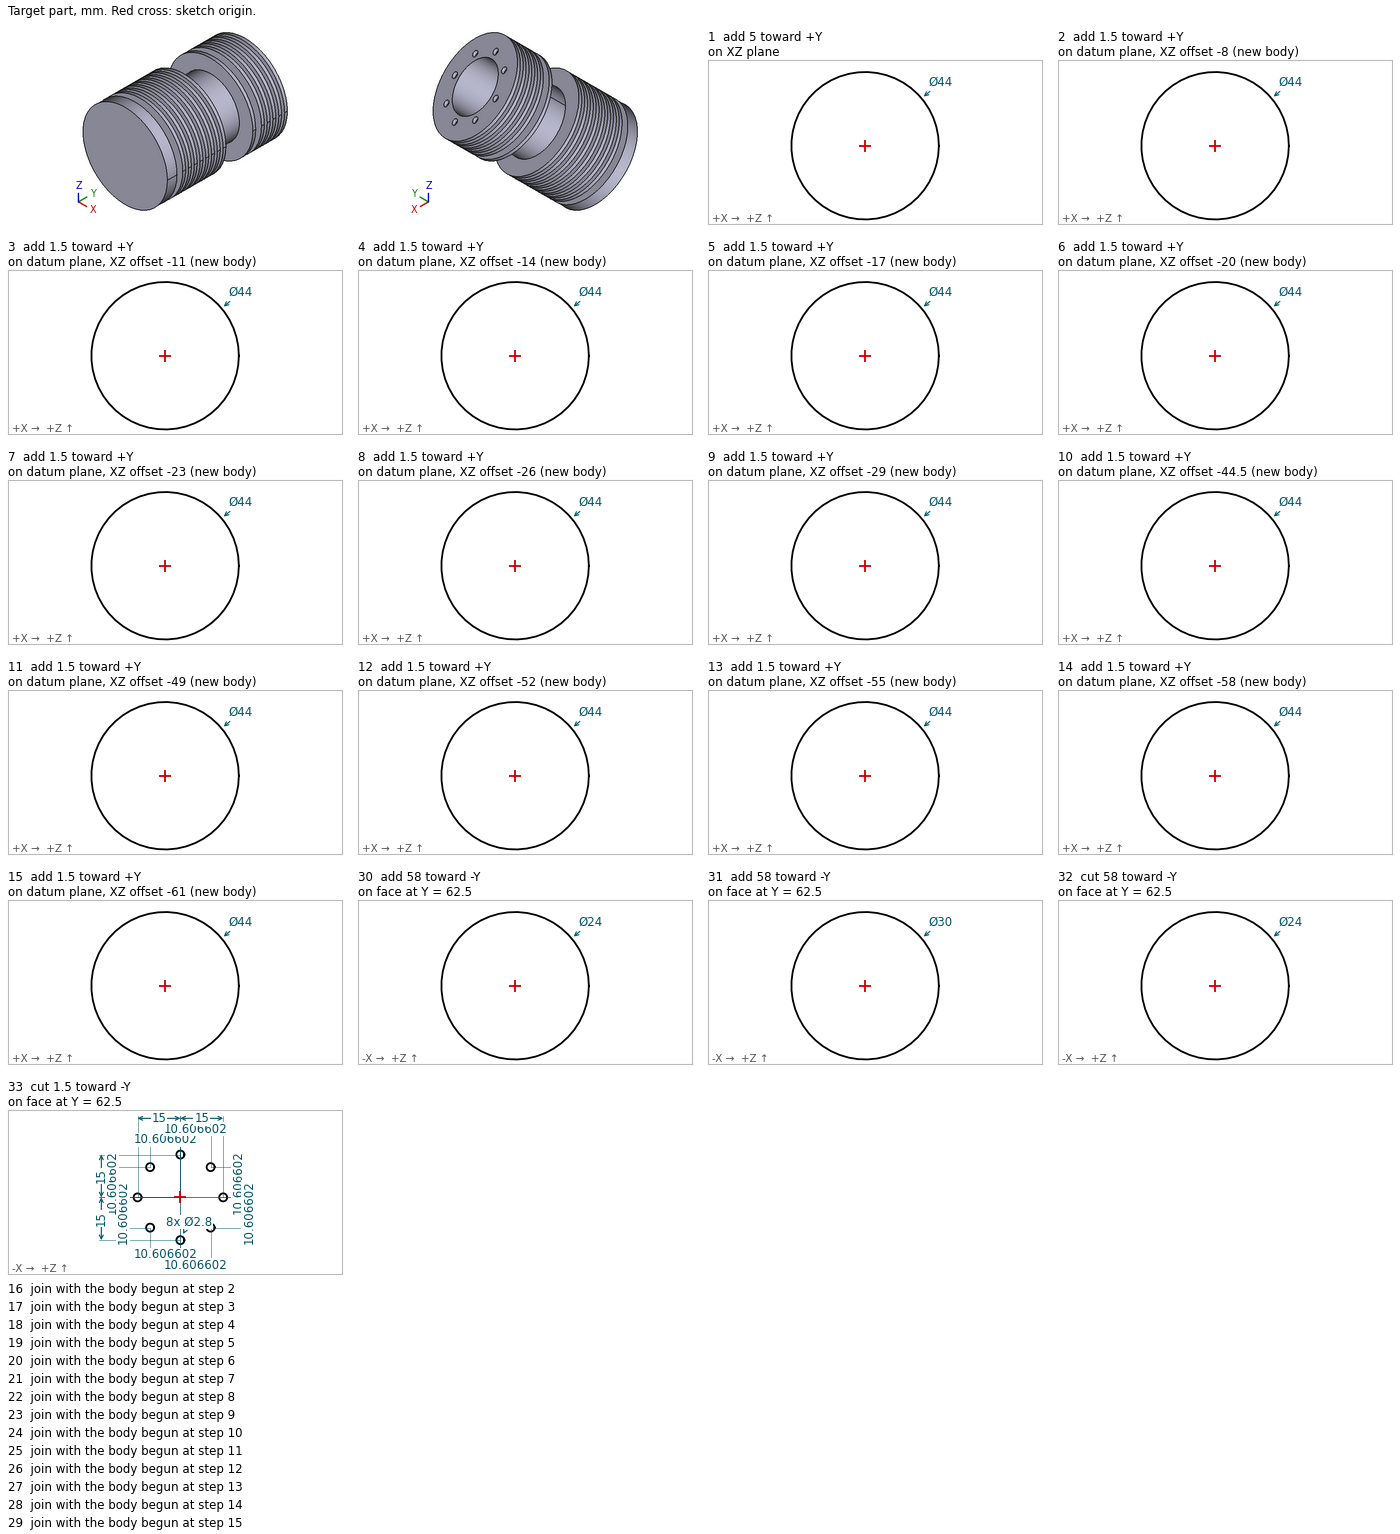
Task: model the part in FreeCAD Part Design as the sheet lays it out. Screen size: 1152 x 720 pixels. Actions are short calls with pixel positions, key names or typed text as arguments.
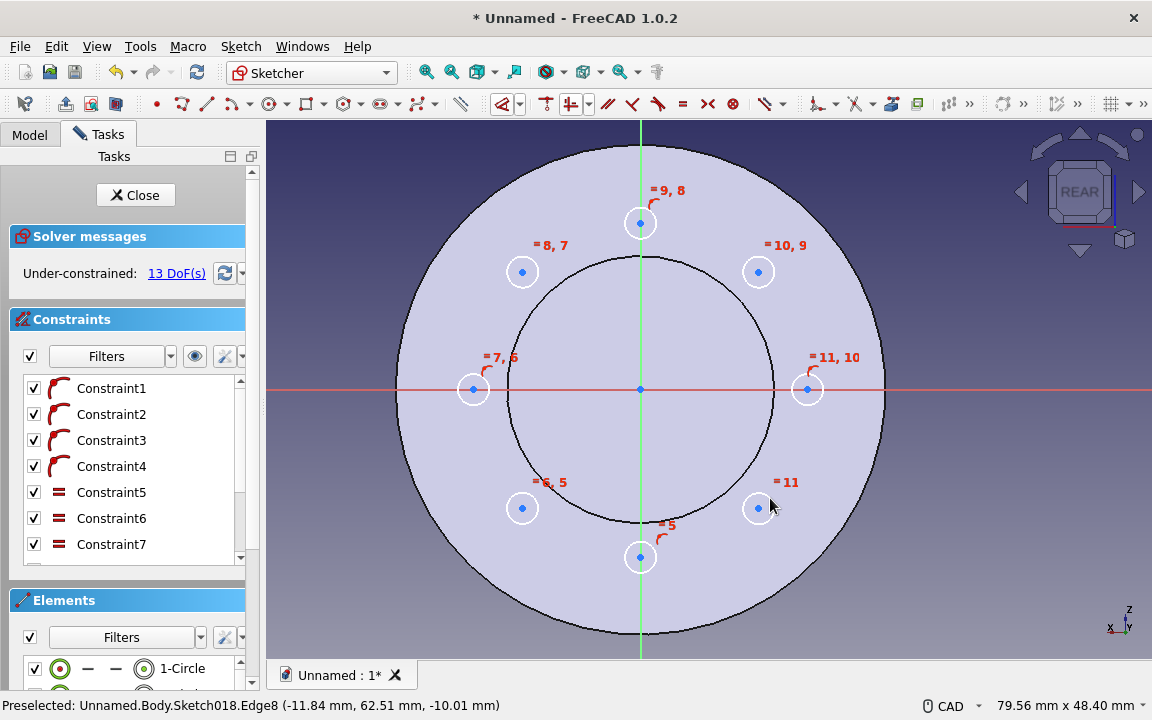
scroll(652, 546, up, 2)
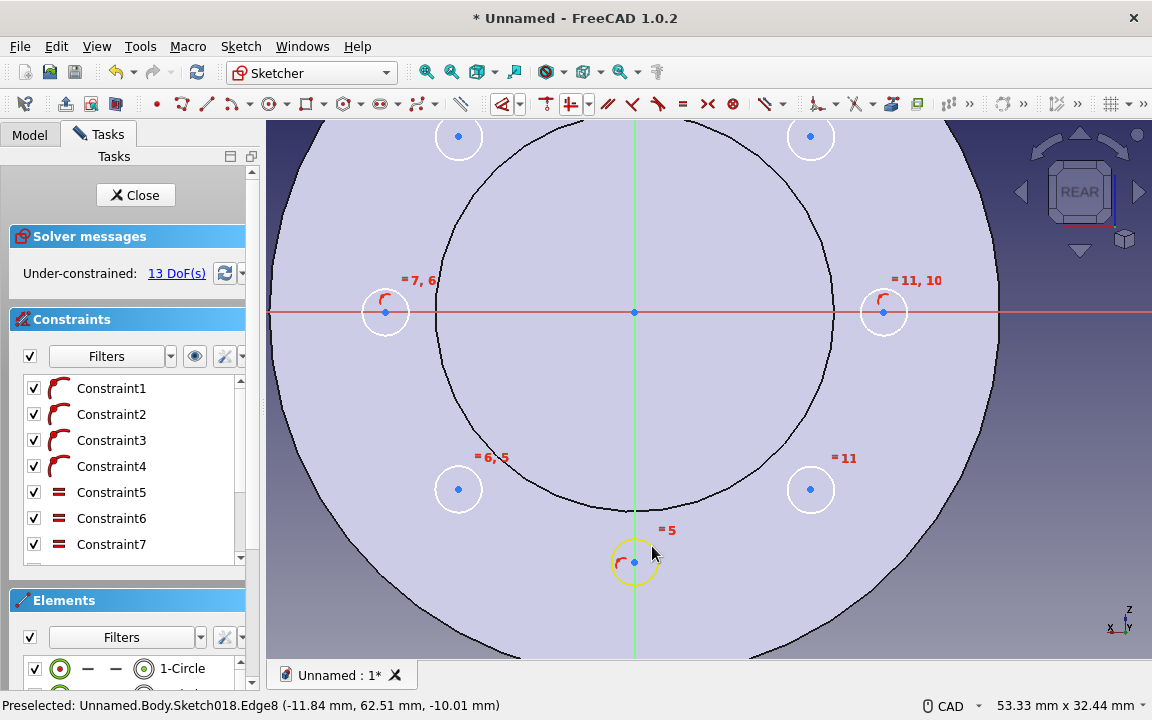
click(651, 546)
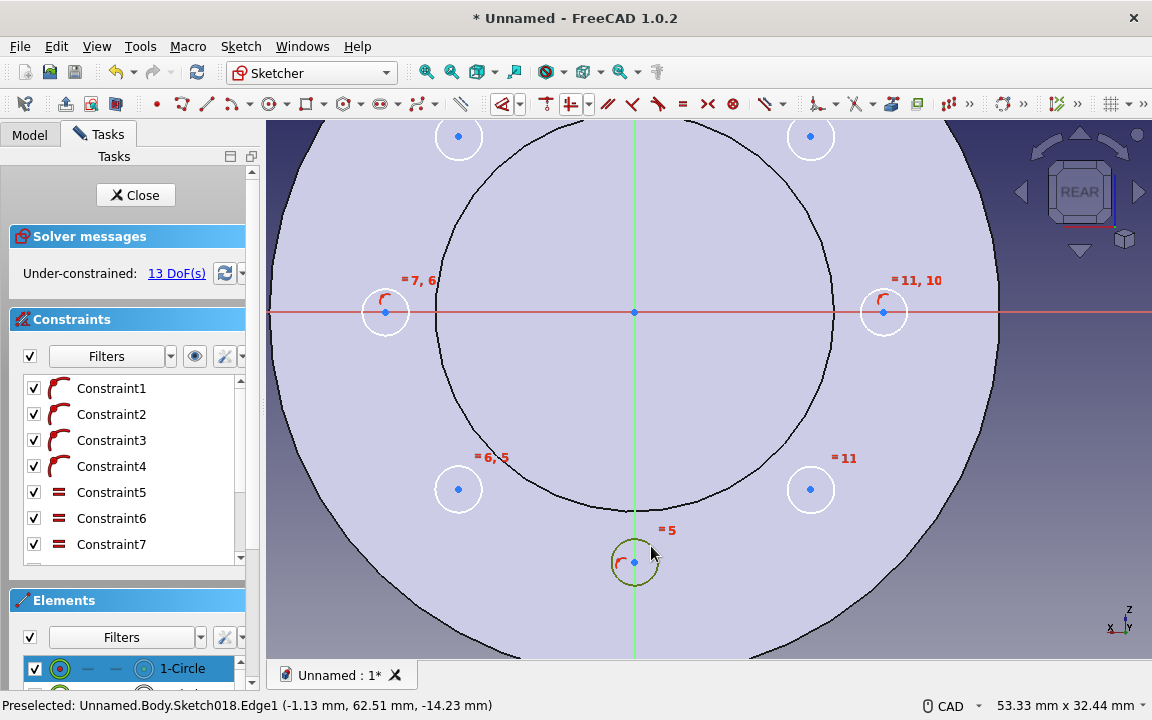
click(520, 104)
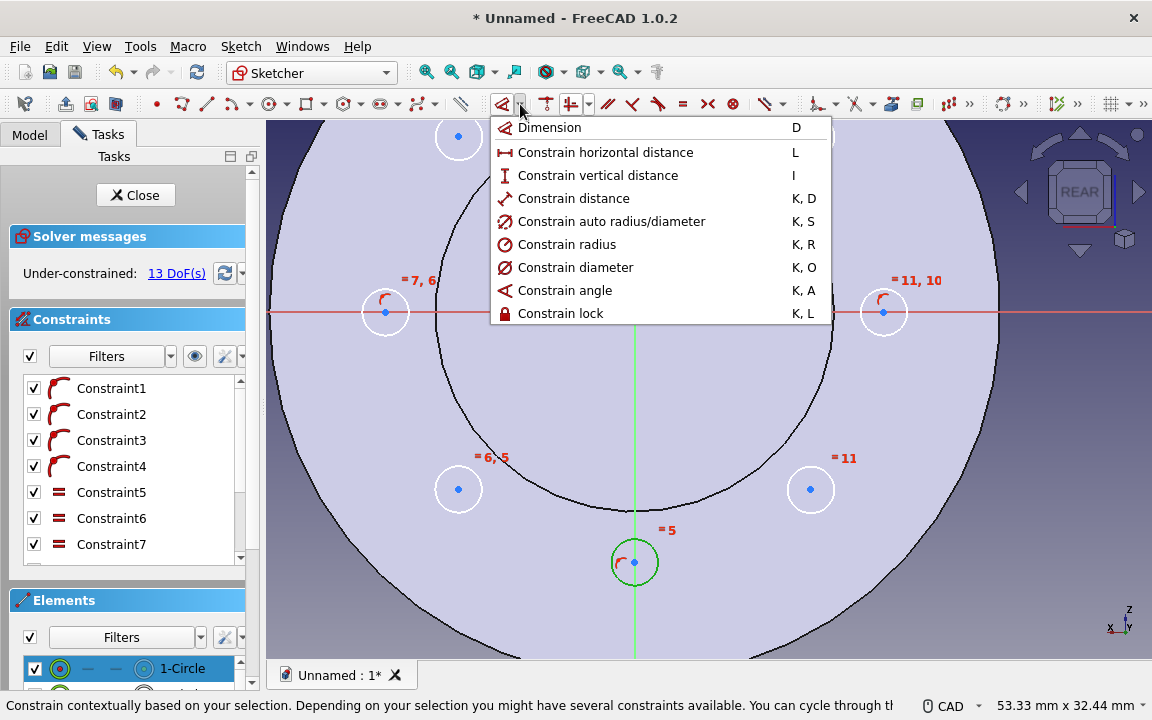
click(661, 268)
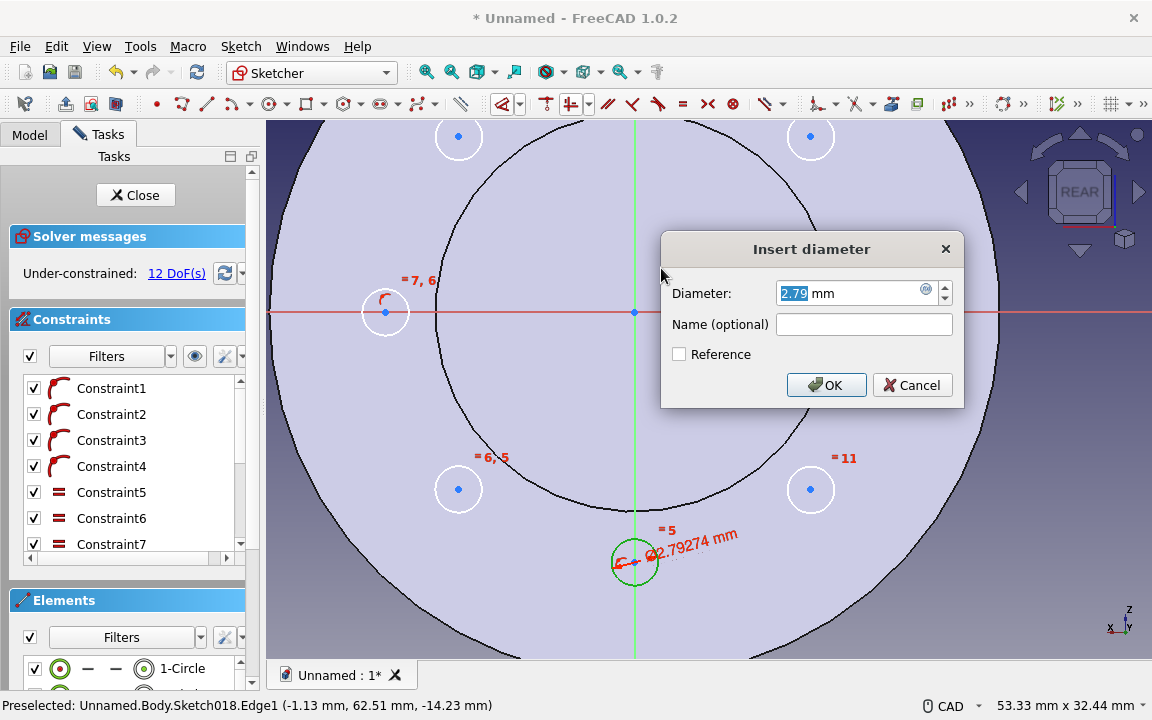
text(2.8)
key(Return)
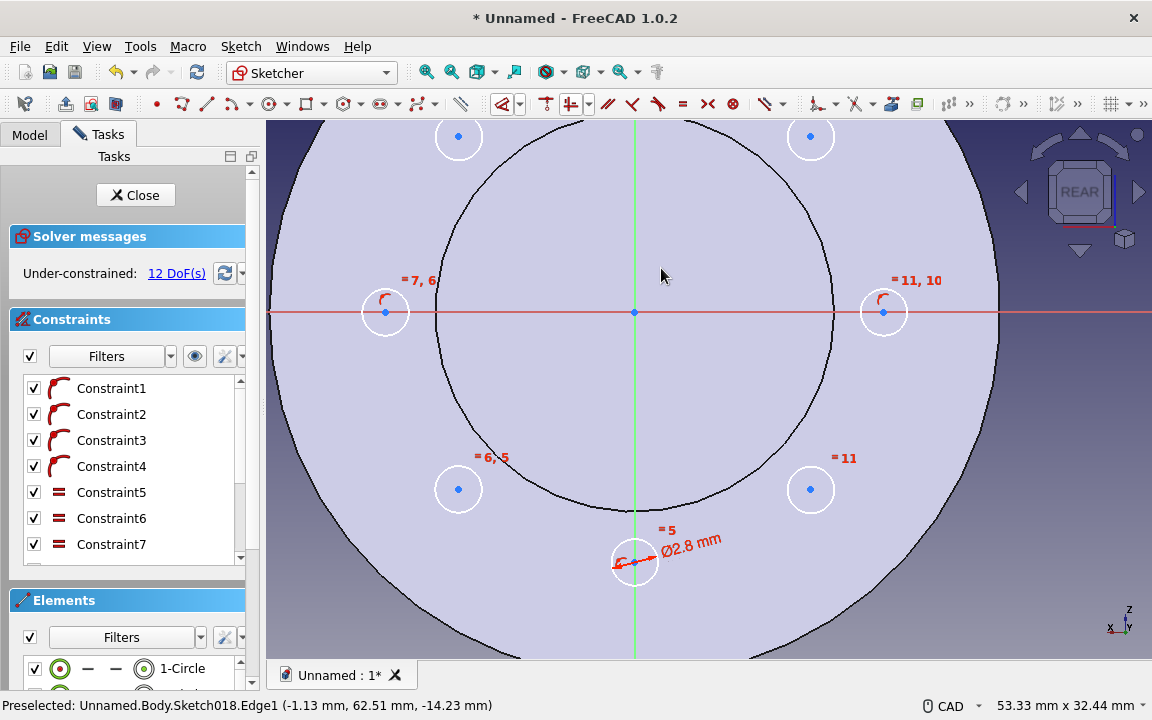
click(635, 562)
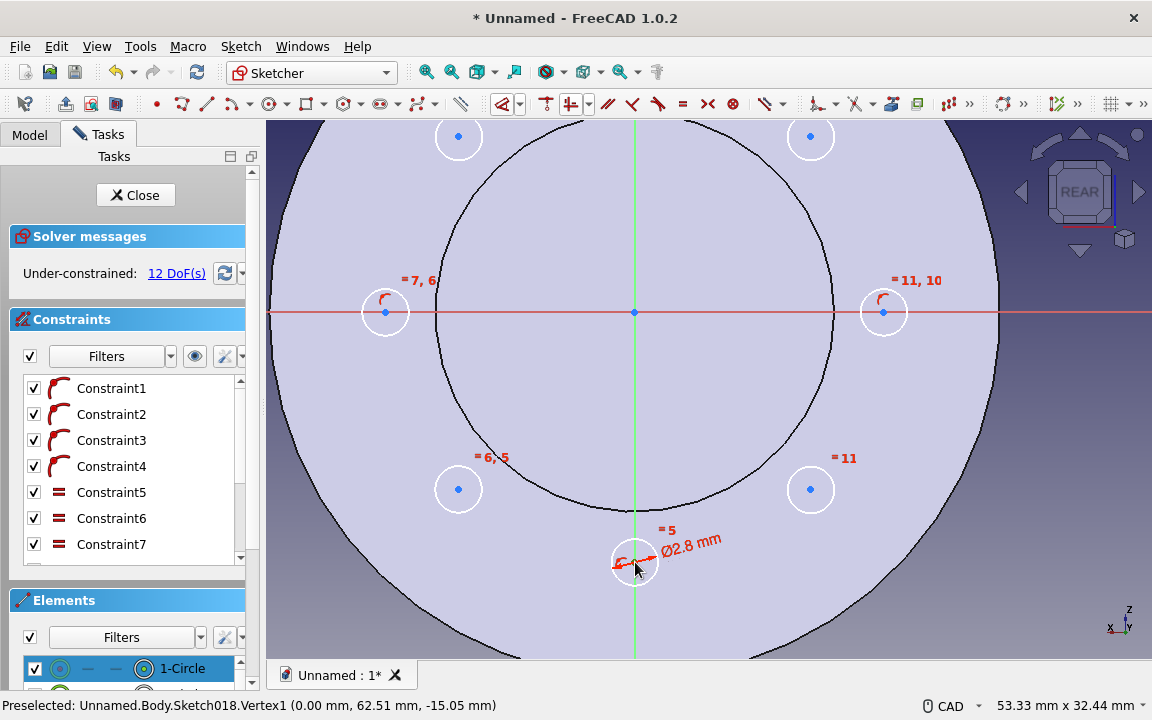
key(i)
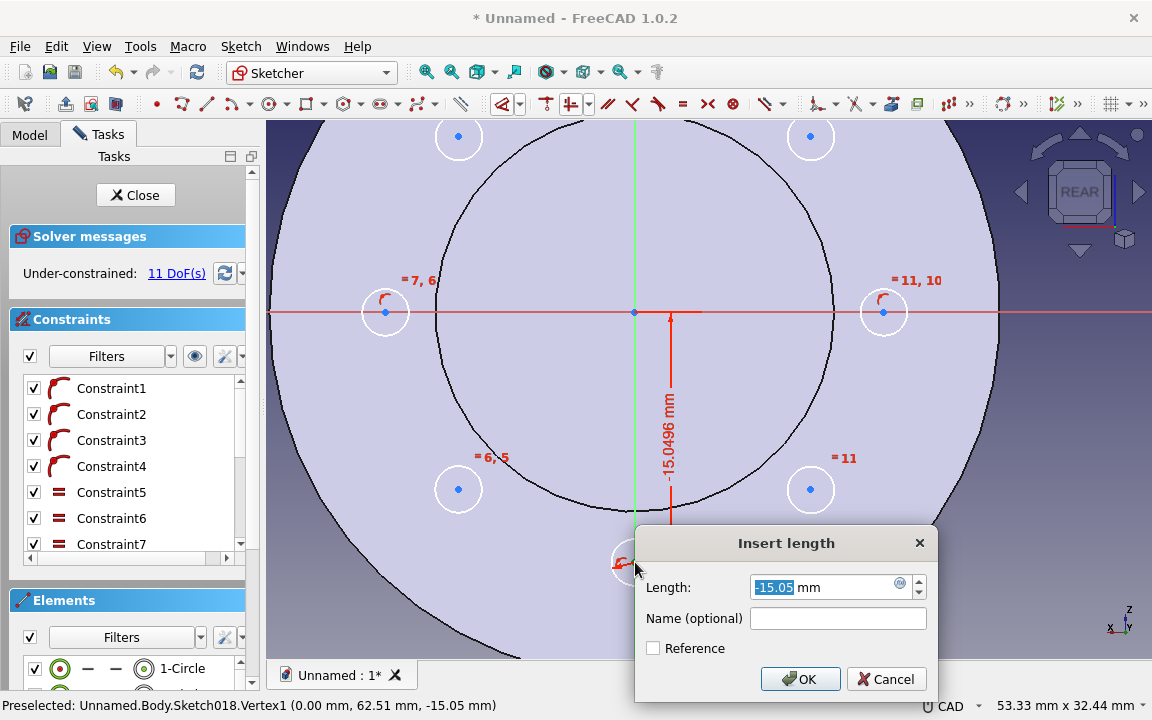
text(-15)
key(Return)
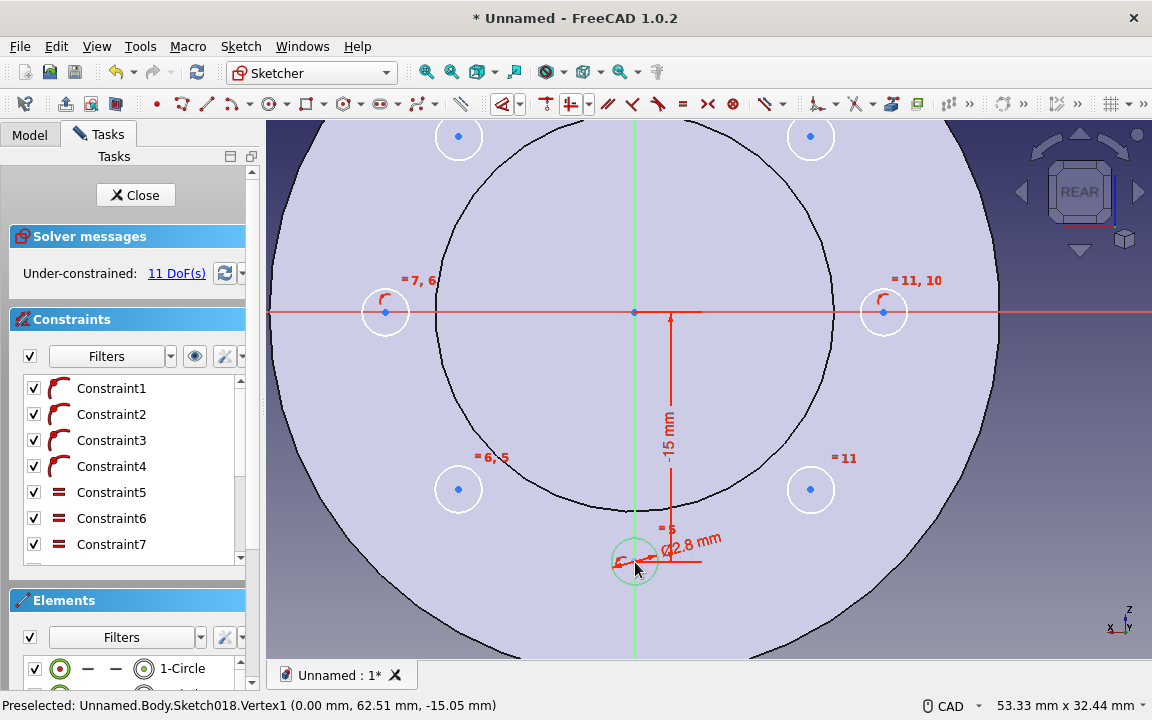
click(386, 312)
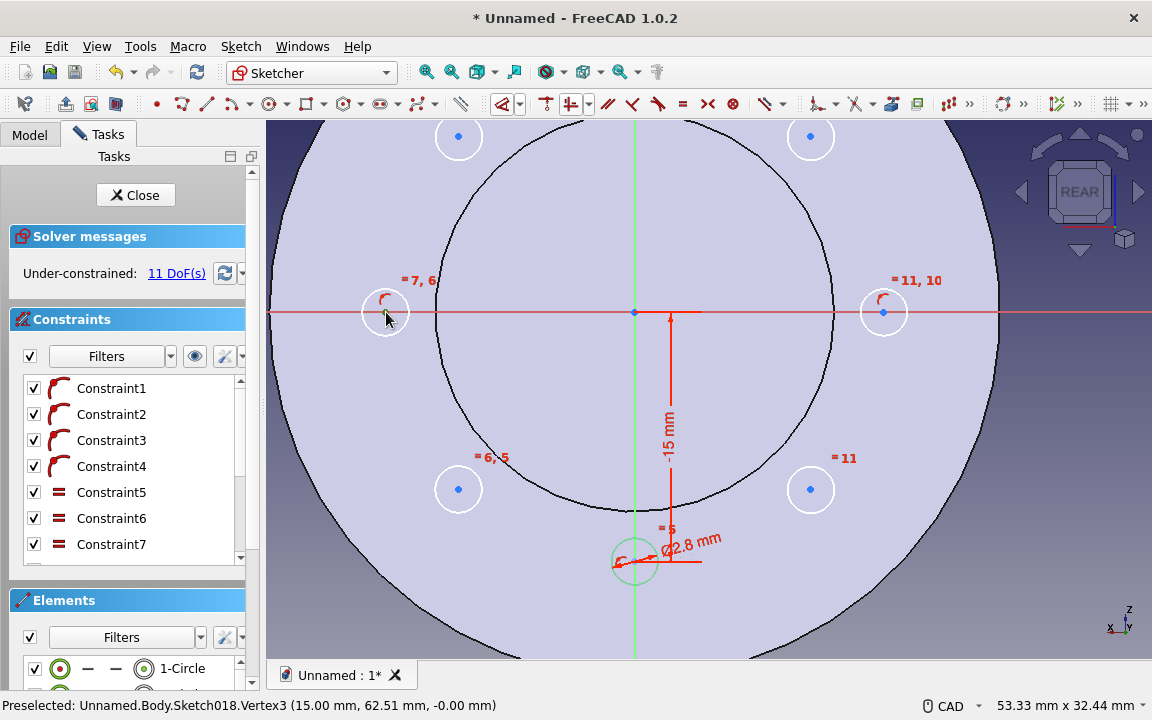
click(520, 104)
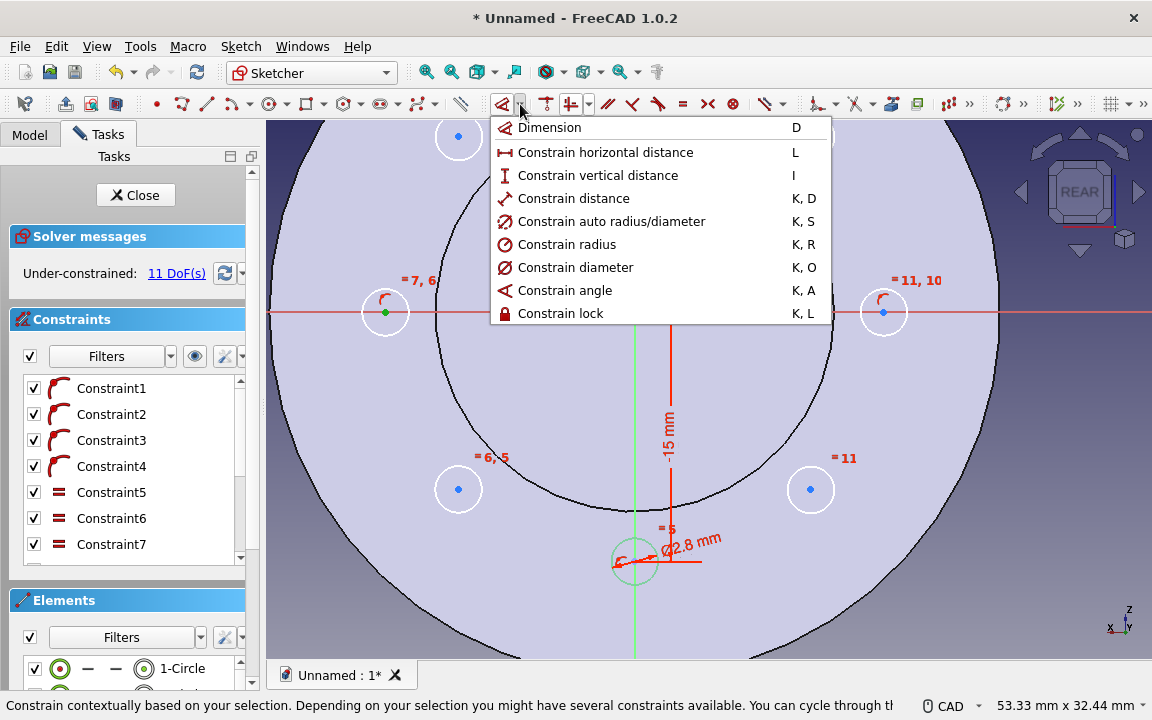
click(661, 152)